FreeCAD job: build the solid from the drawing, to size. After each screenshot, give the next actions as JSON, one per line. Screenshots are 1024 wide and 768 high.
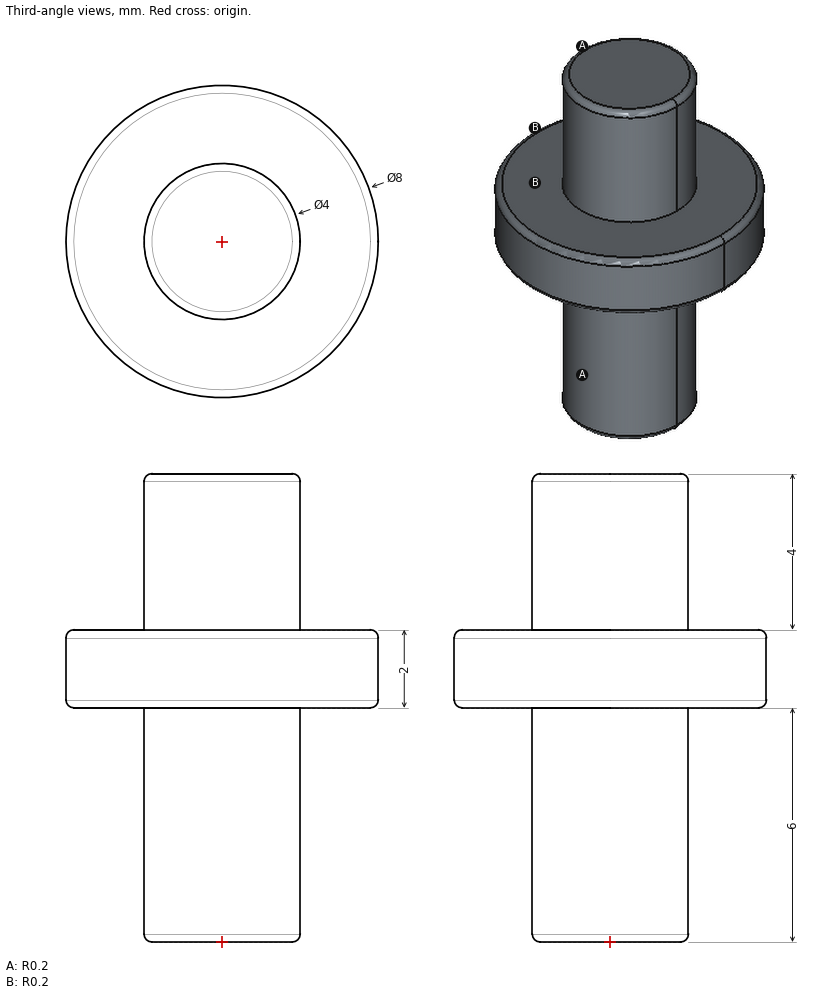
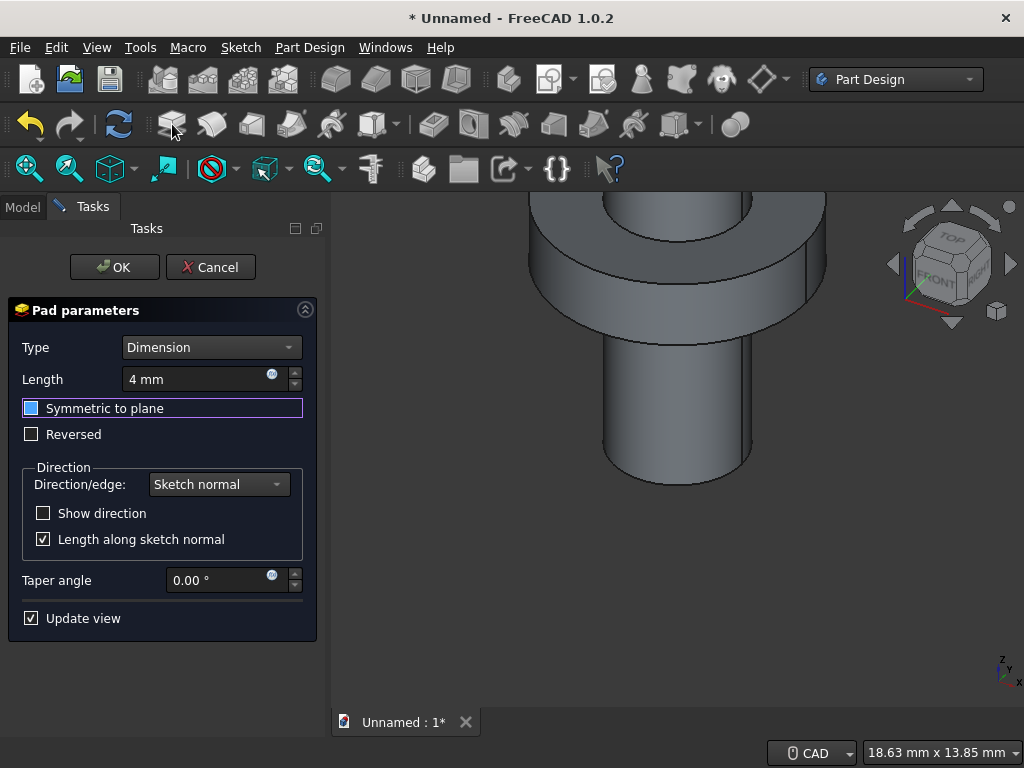
{"action": "left_click", "coordinate": [115, 267]}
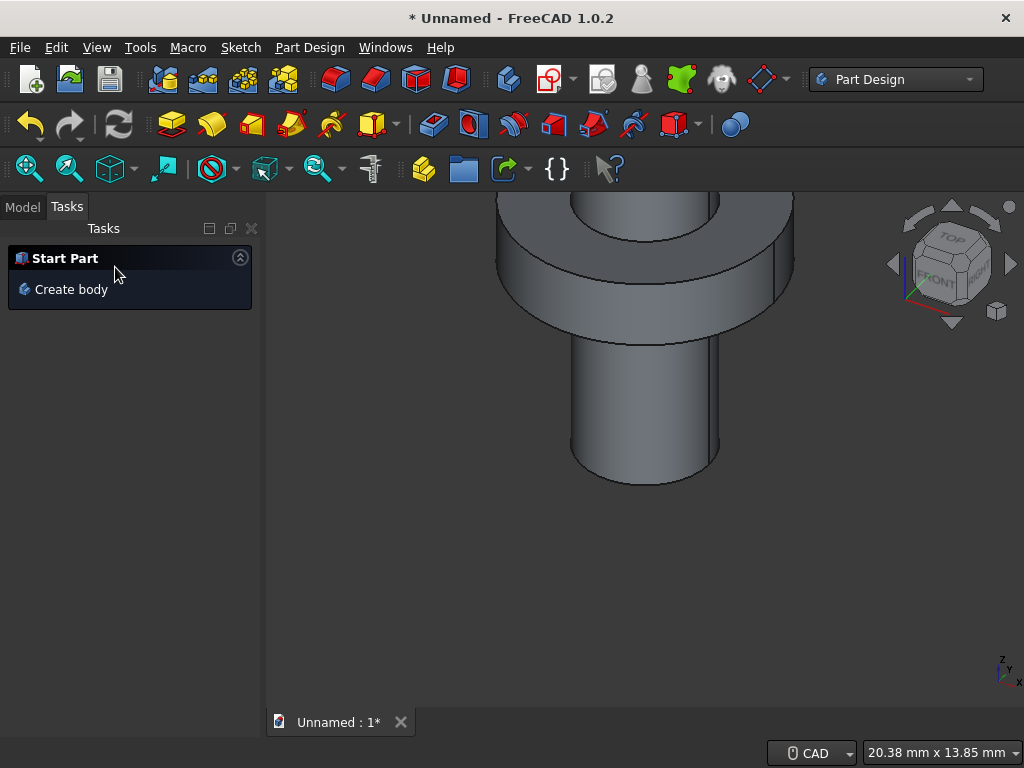
{"action": "left_click", "coordinate": [30, 170]}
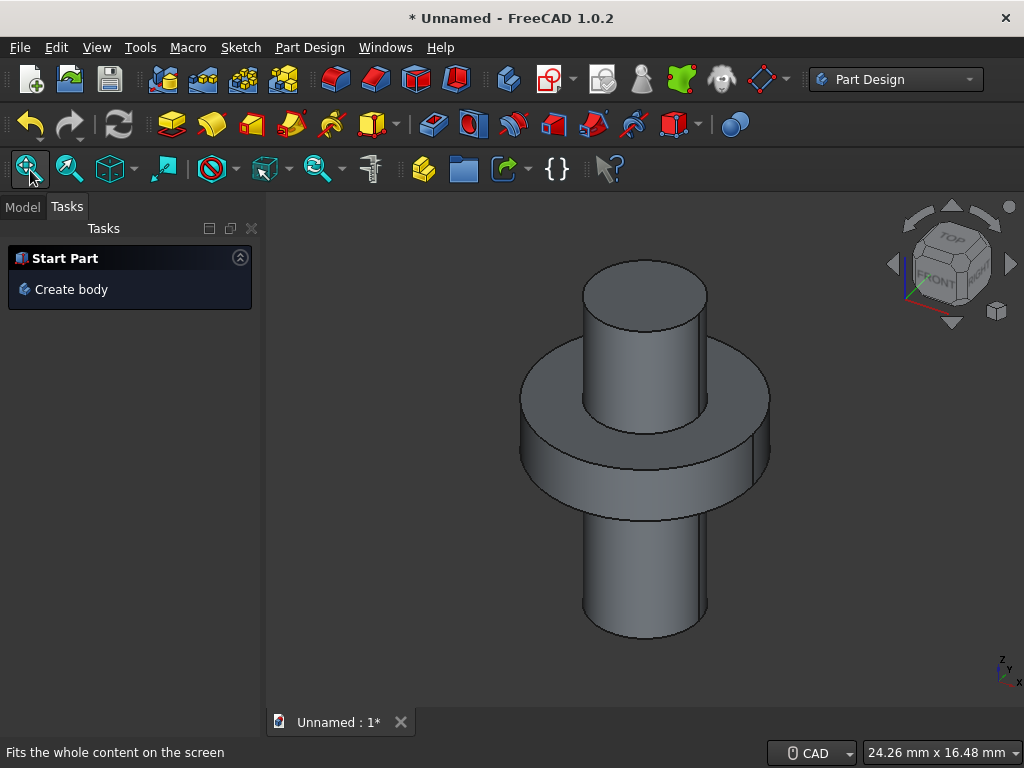
{"action": "left_click", "coordinate": [583, 299]}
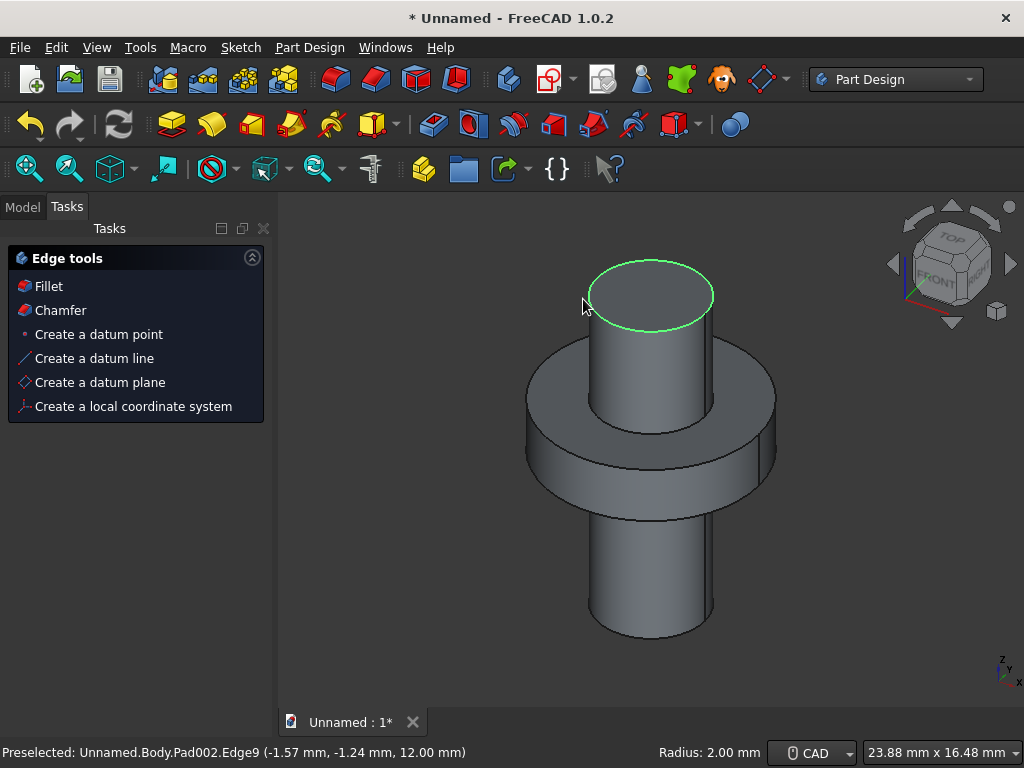
{"action": "key", "text": "0"}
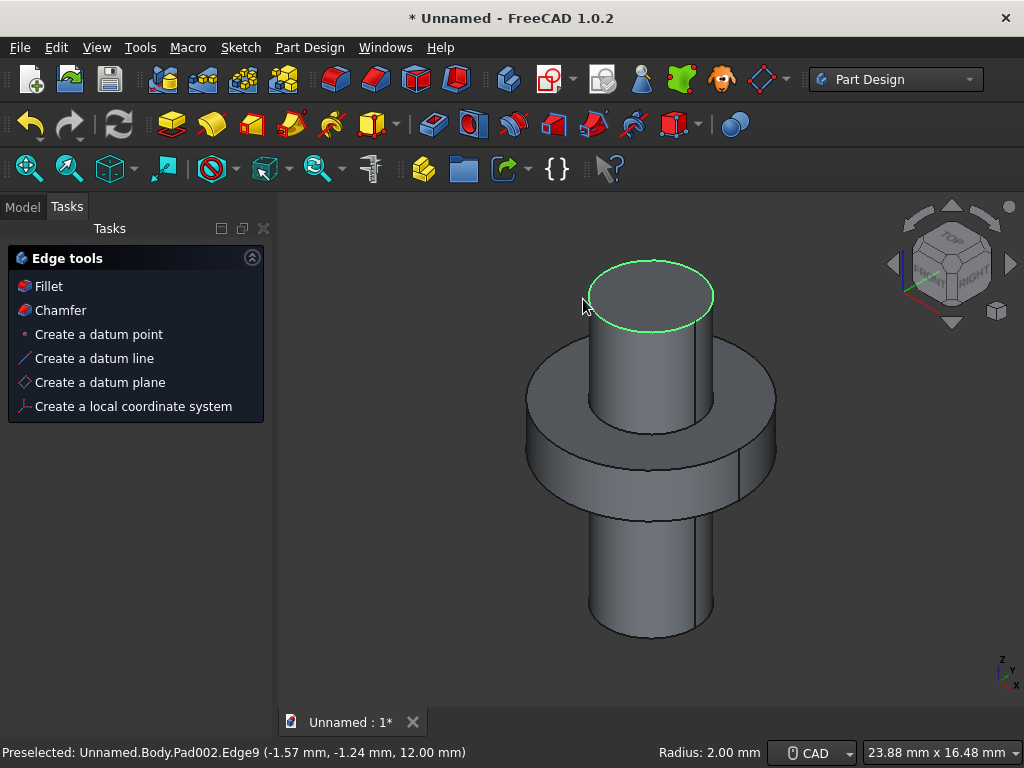
{"action": "key", "text": "2"}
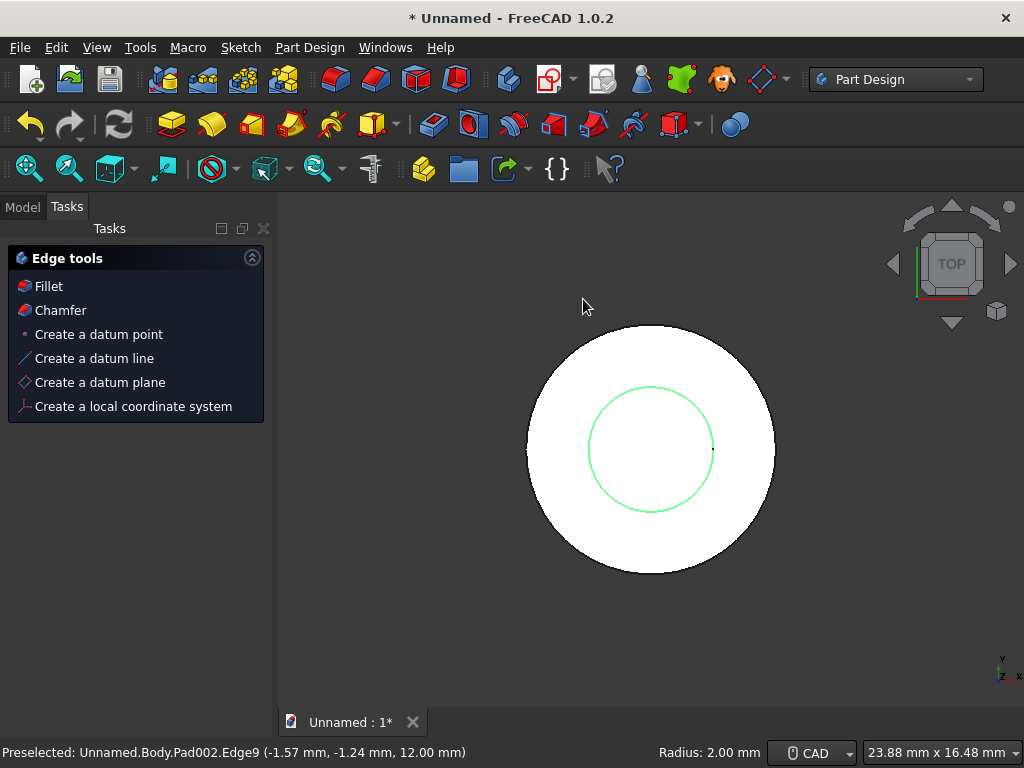
{"action": "key", "text": "1"}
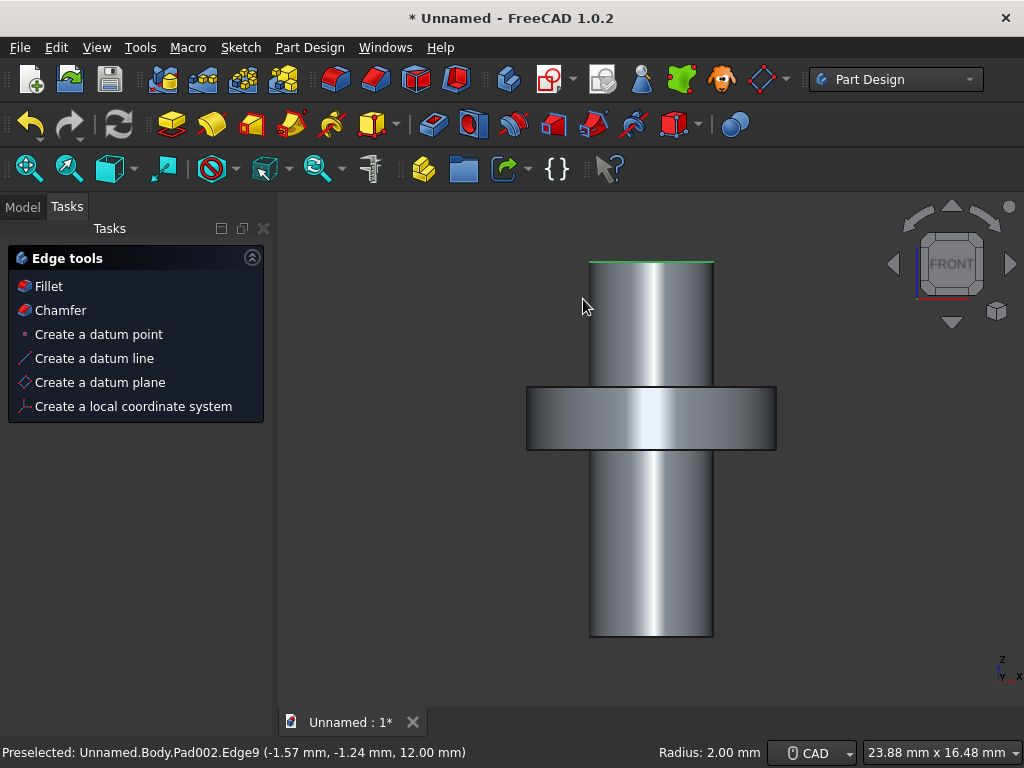
{"action": "left_click", "coordinate": [589, 636], "text": "ctrl"}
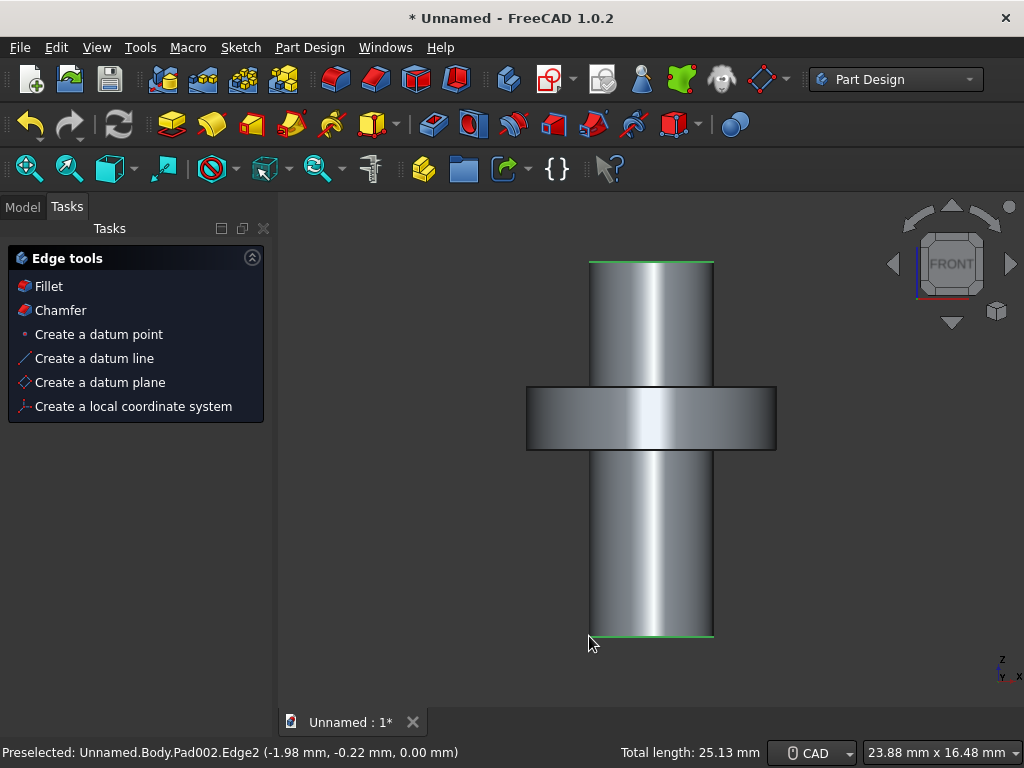
{"action": "left_click", "coordinate": [336, 80]}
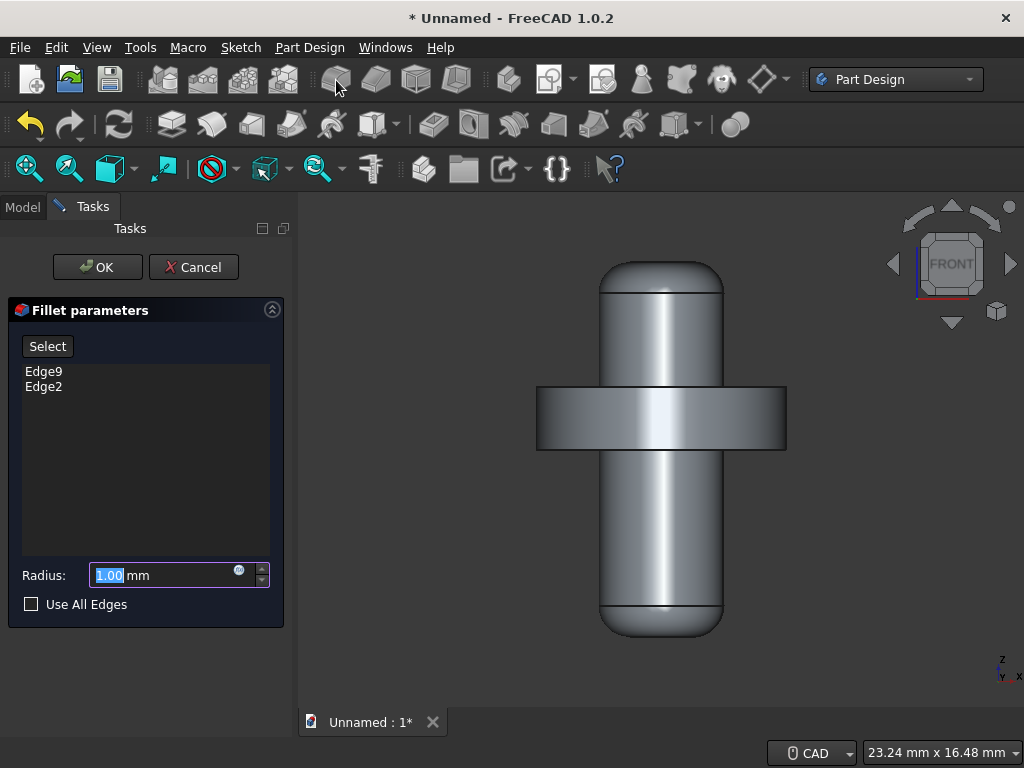
{"action": "type", "text": "0.2"}
{"action": "key", "text": "Tab"}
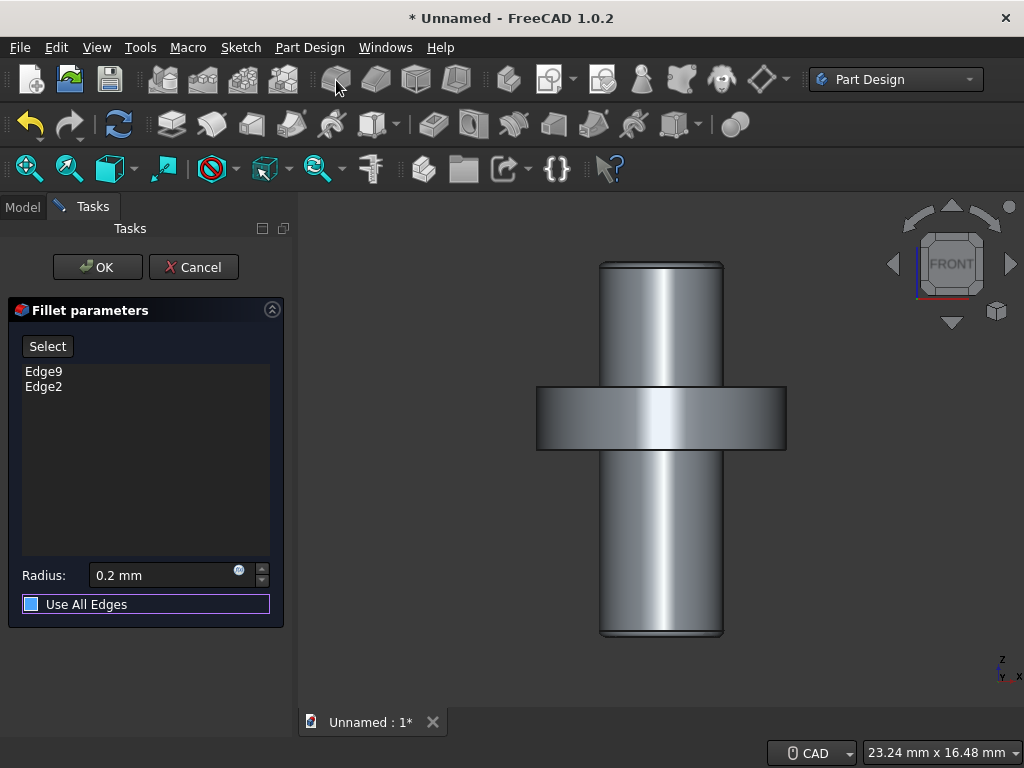
{"action": "left_click", "coordinate": [98, 267]}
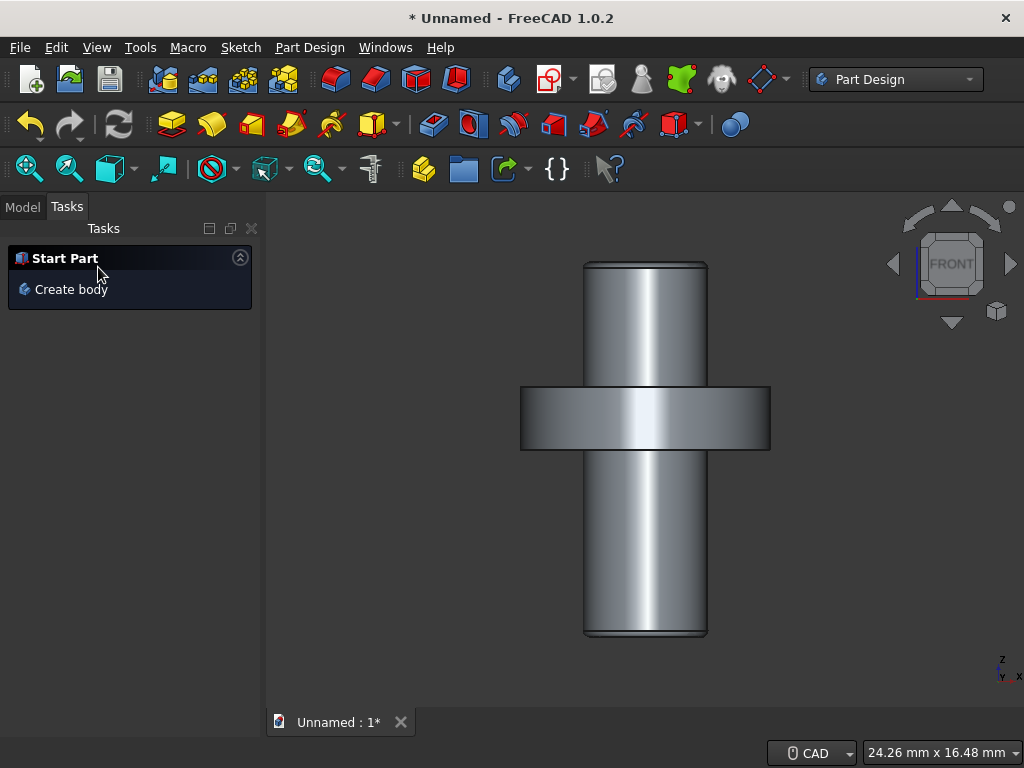
{"action": "left_click", "coordinate": [544, 448]}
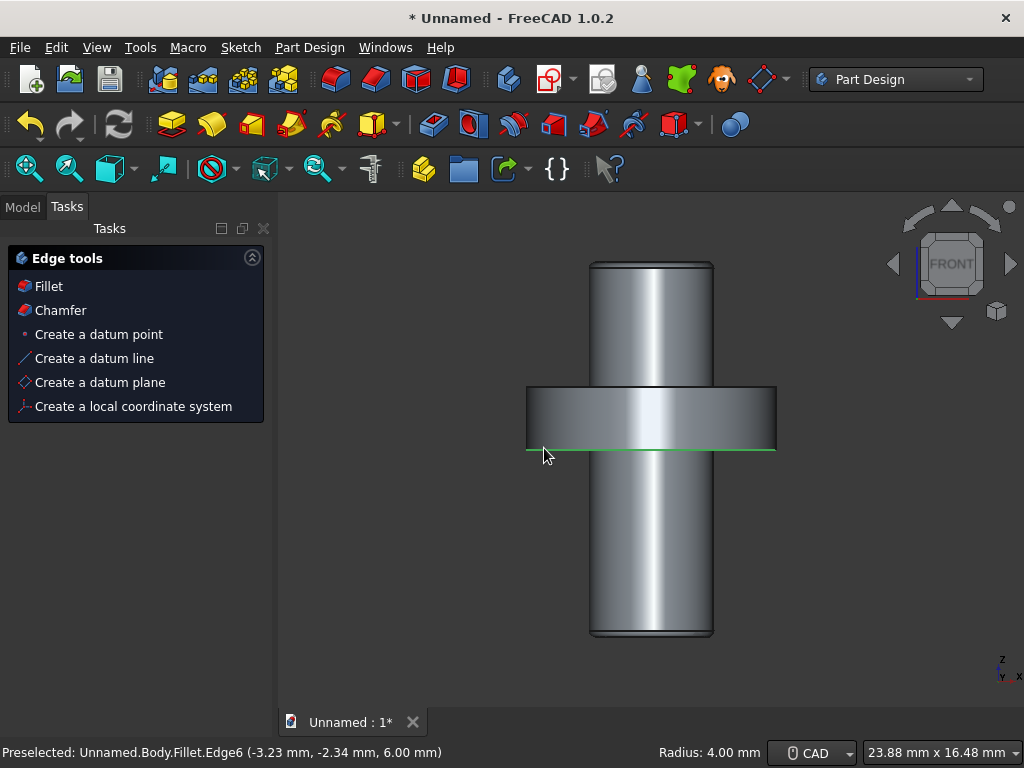
{"action": "left_click", "coordinate": [550, 386], "text": "ctrl"}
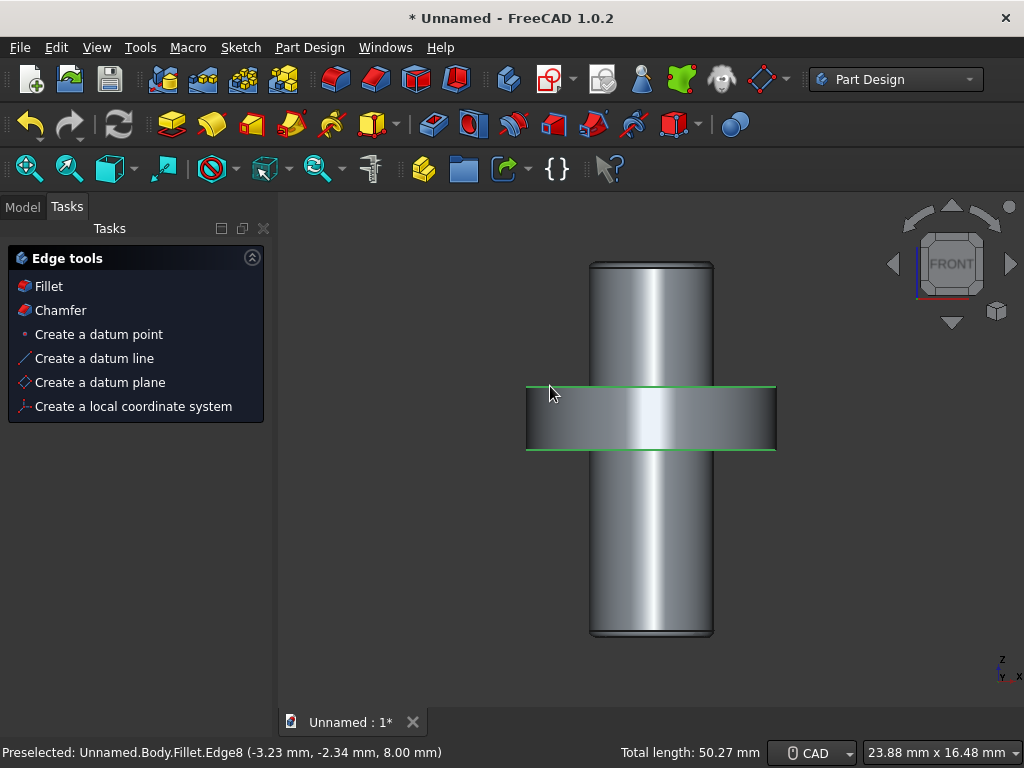
{"action": "left_click", "coordinate": [336, 80]}